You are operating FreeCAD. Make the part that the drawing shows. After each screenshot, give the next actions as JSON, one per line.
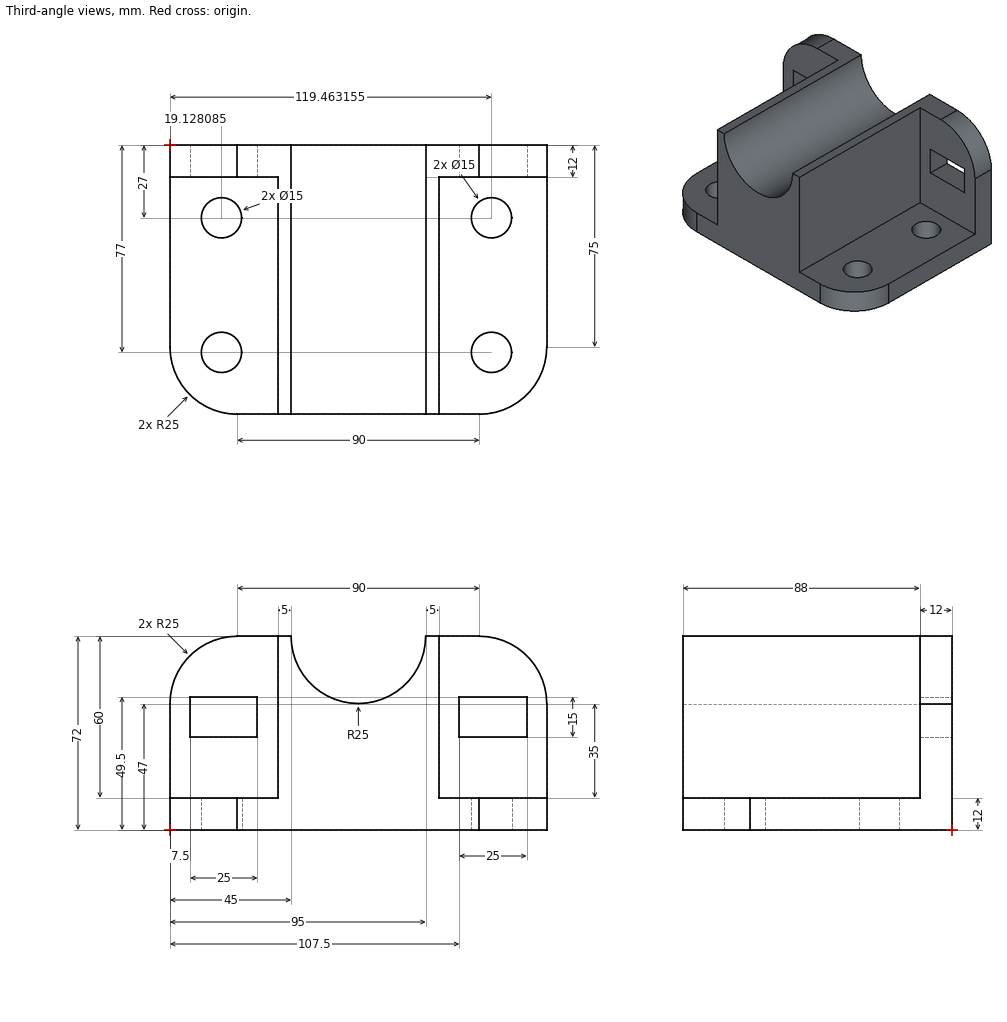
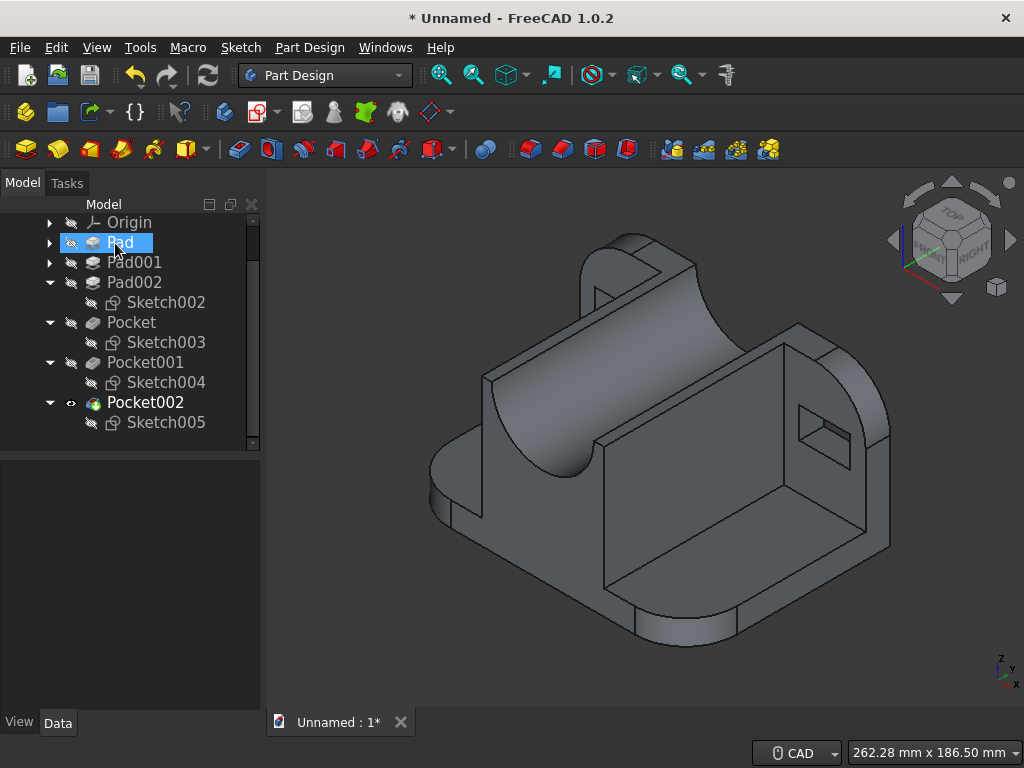
{"action": "key", "text": "2"}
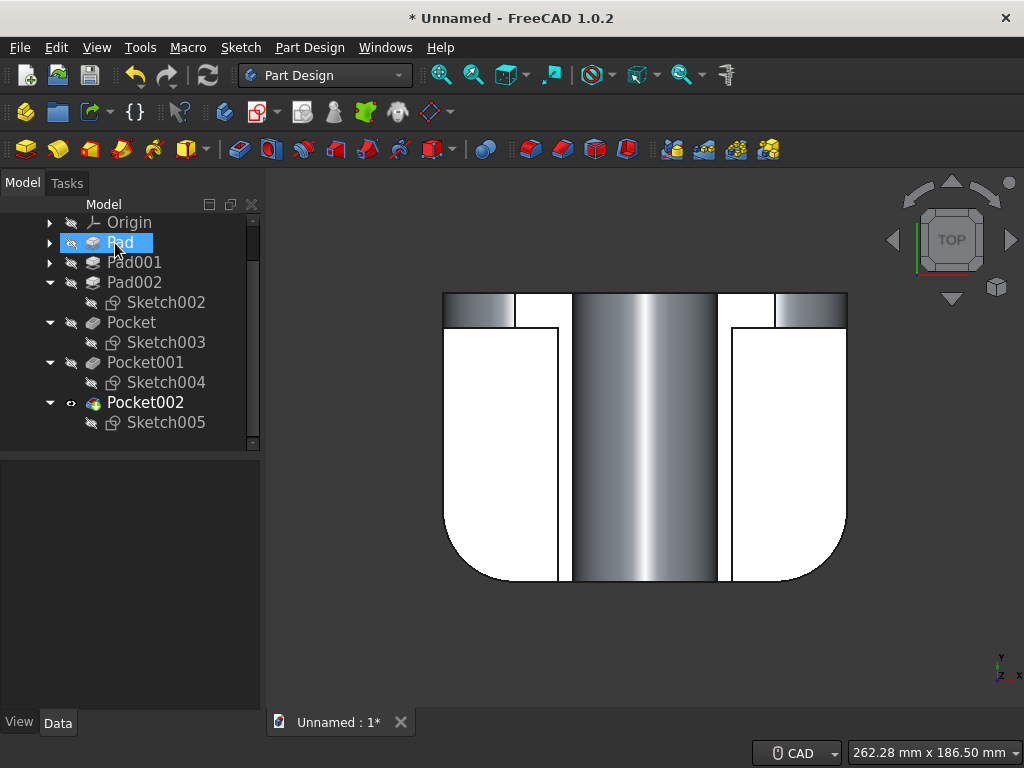
{"action": "left_click", "coordinate": [500, 418]}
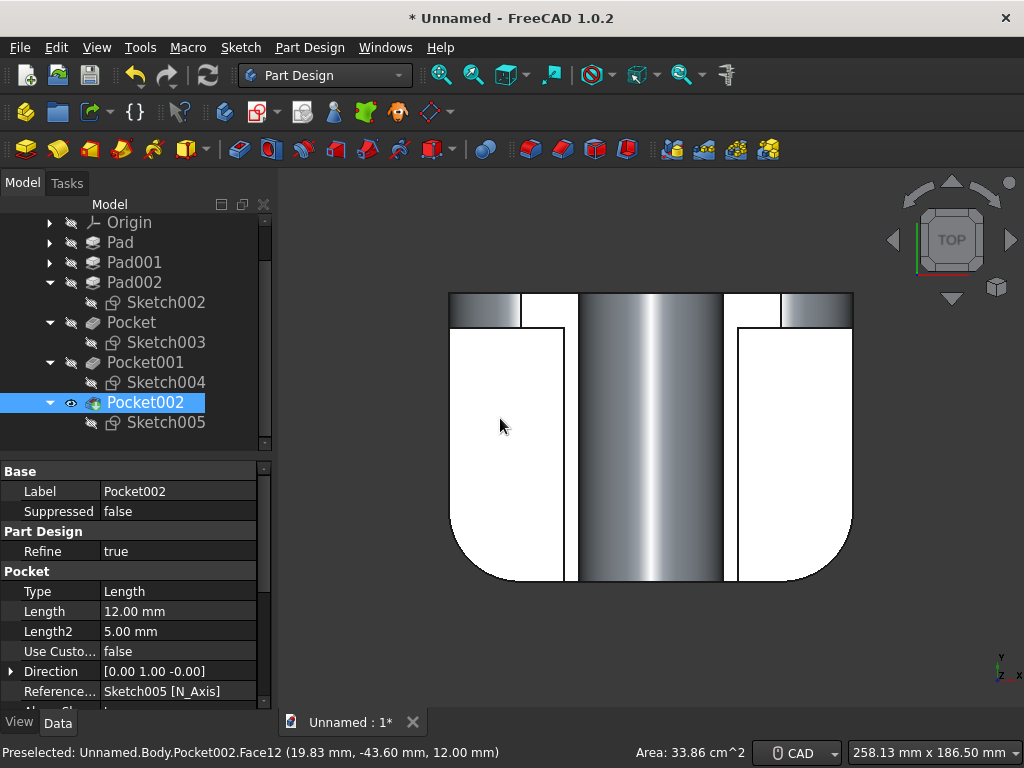
{"action": "left_click", "coordinate": [258, 112]}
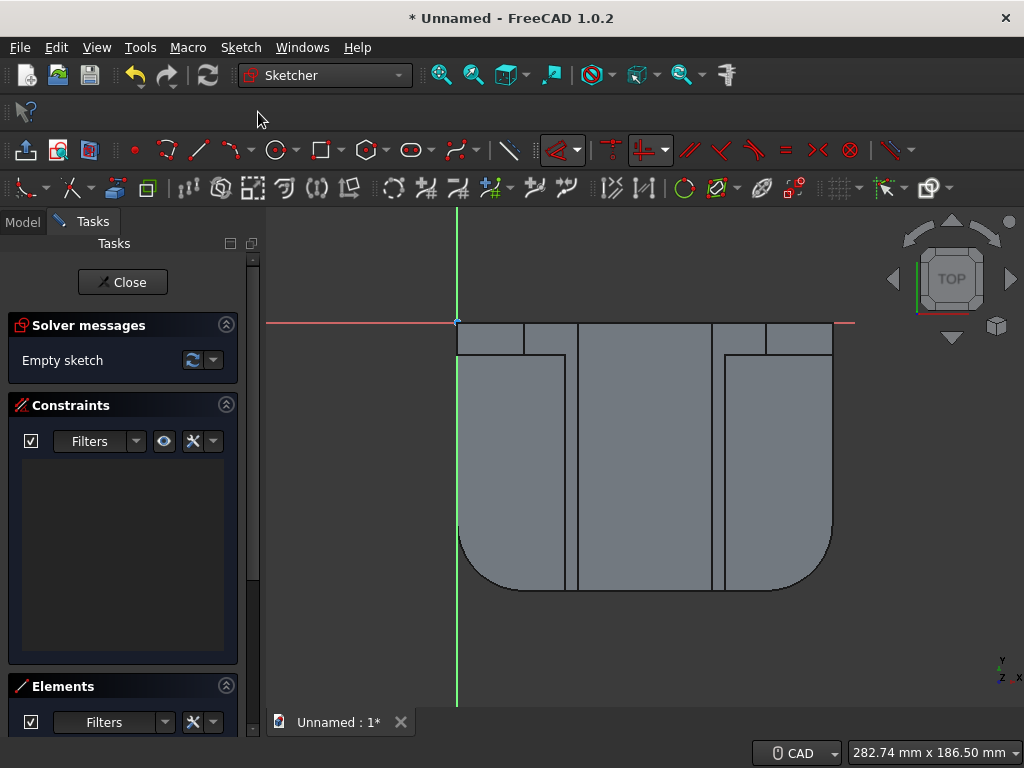
{"action": "key", "text": "q s"}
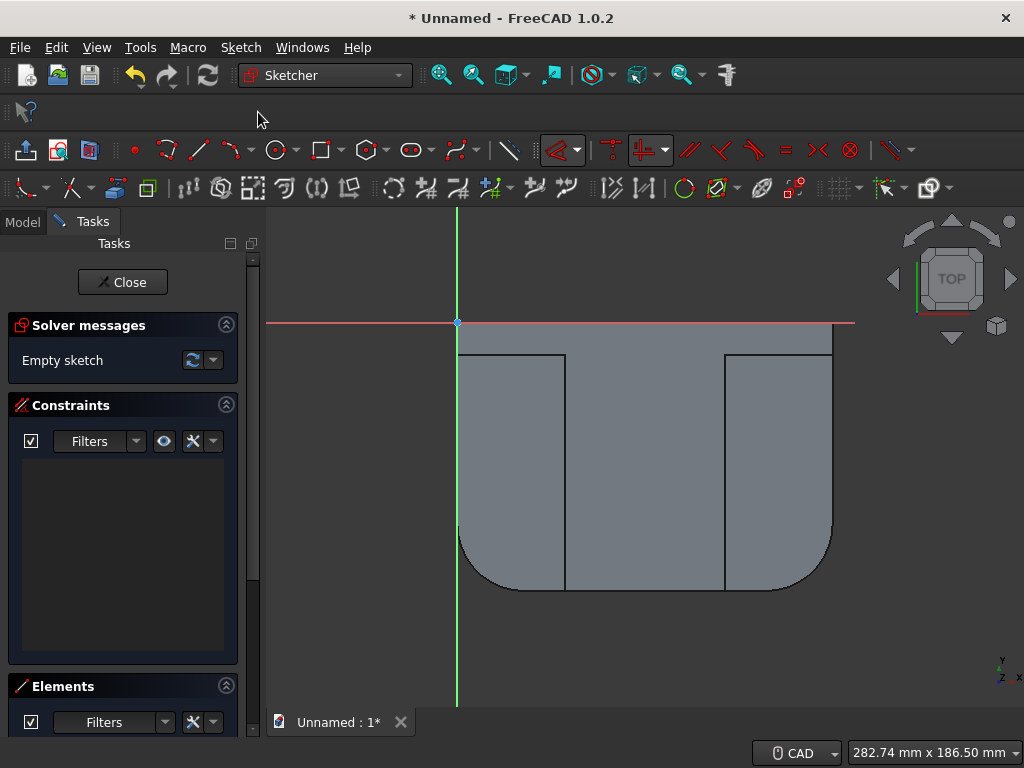
{"action": "key", "text": "g c"}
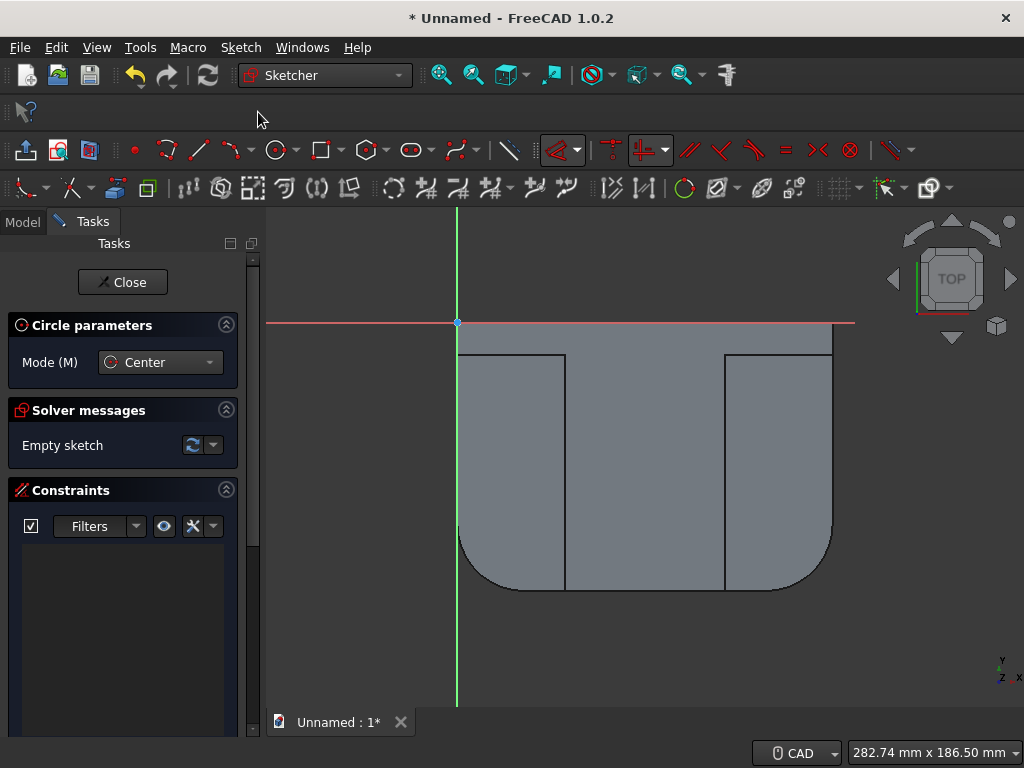
{"action": "left_click", "coordinate": [778, 395]}
{"action": "left_click", "coordinate": [792, 381]}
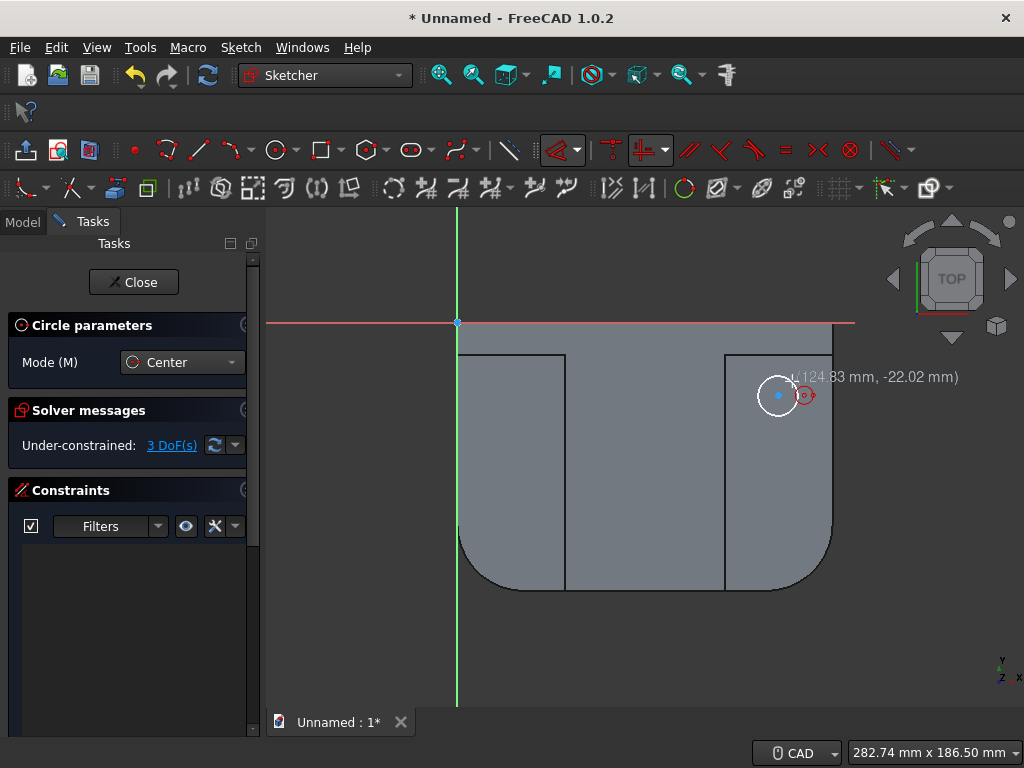
{"action": "left_click", "coordinate": [778, 529]}
{"action": "left_click", "coordinate": [792, 515]}
{"action": "key", "text": "Escape"}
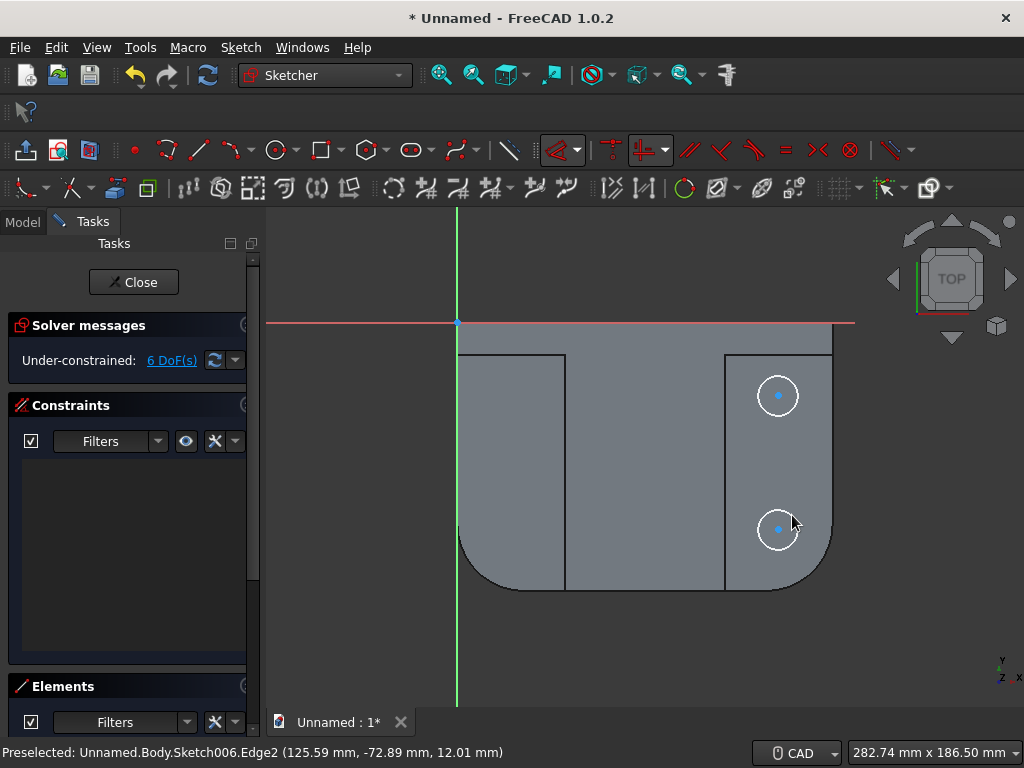
{"action": "left_click", "coordinate": [792, 382]}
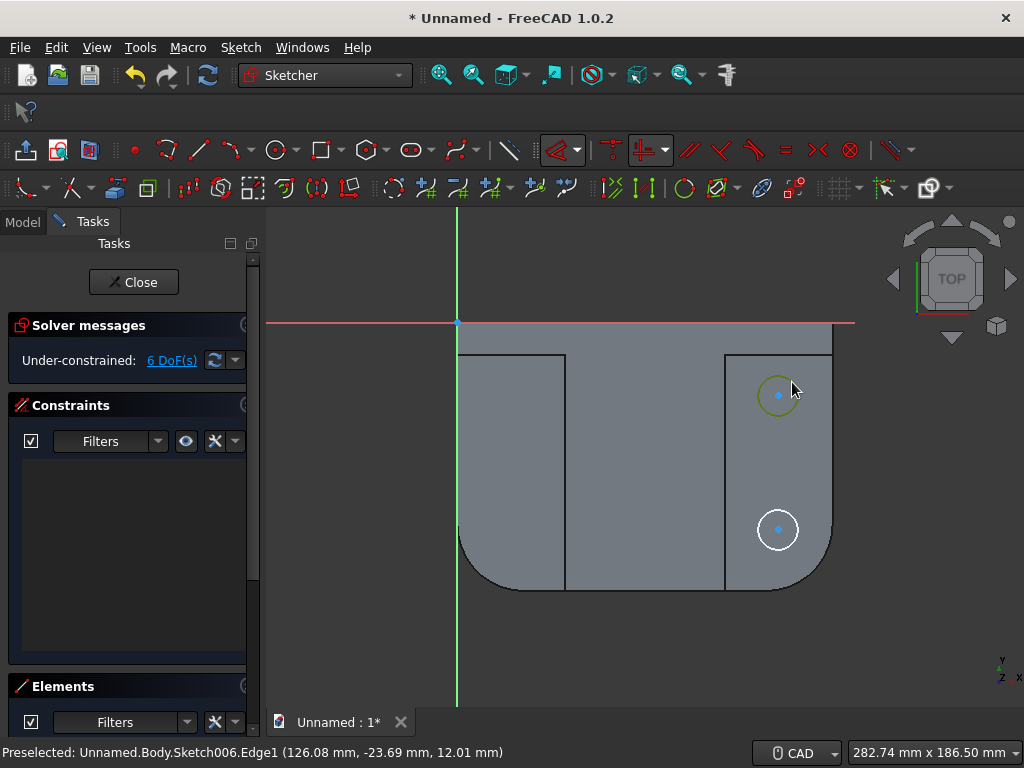
{"action": "left_click", "coordinate": [792, 516]}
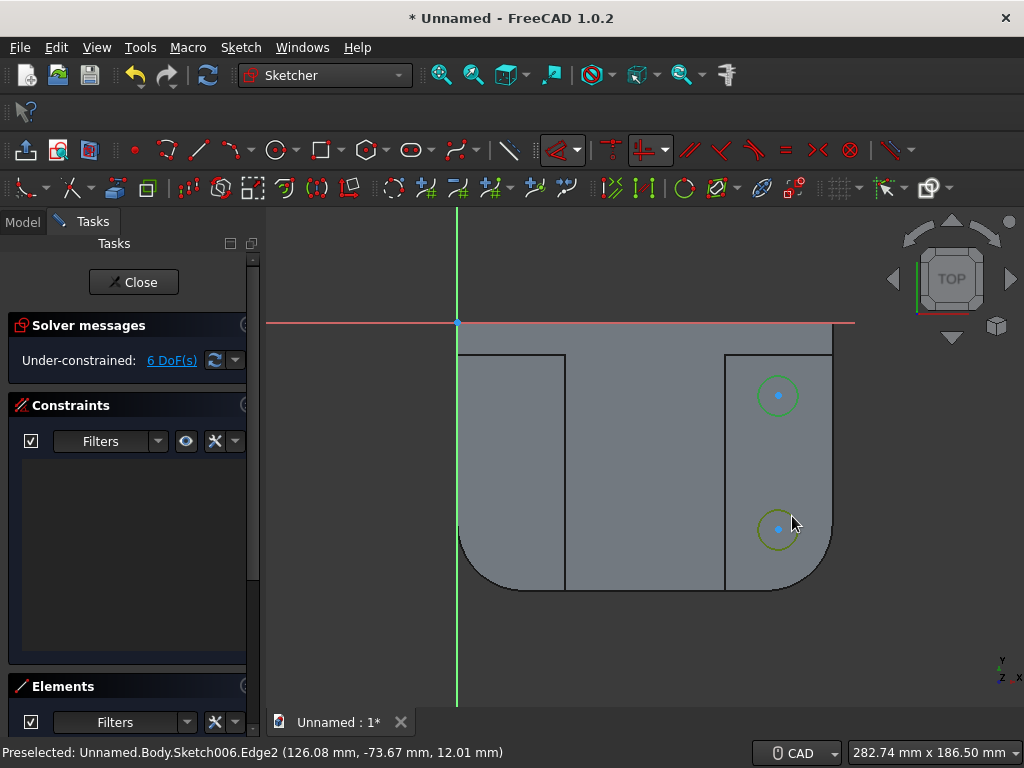
{"action": "key", "text": "e"}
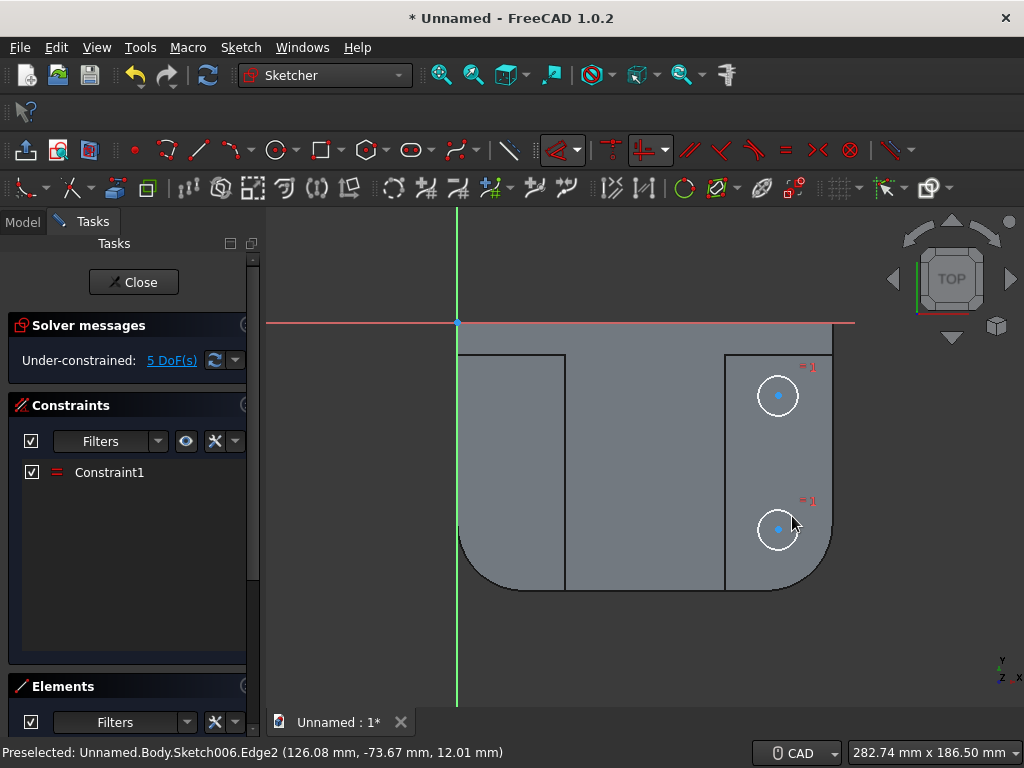
{"action": "left_click", "coordinate": [778, 396]}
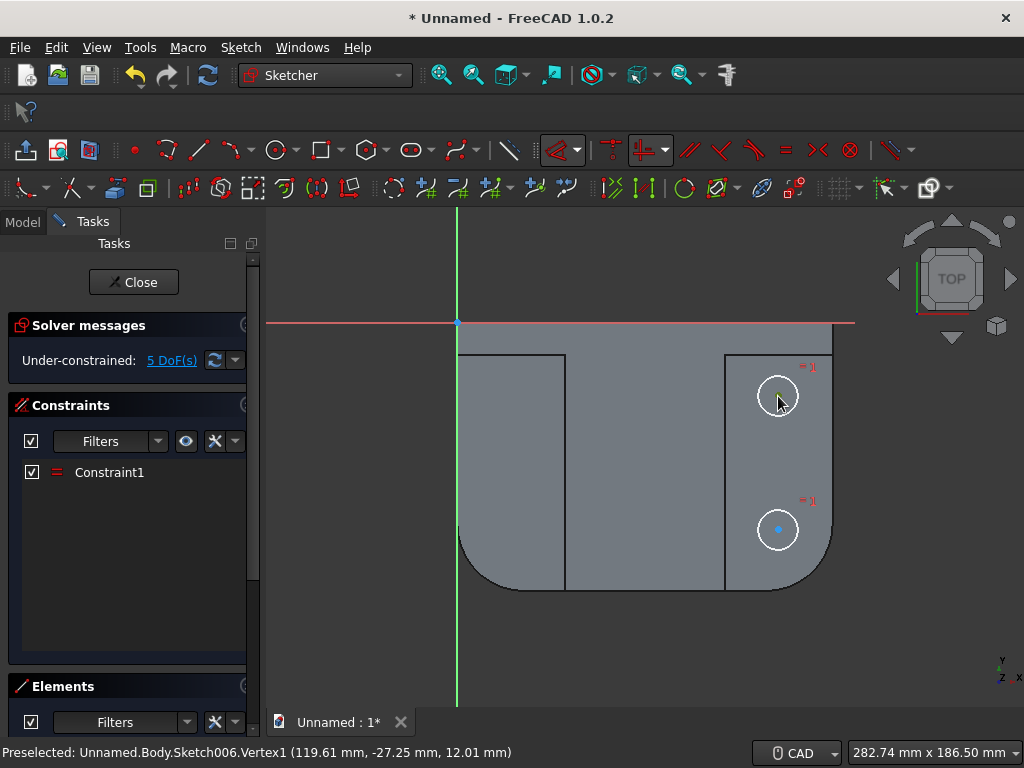
{"action": "left_click", "coordinate": [778, 530]}